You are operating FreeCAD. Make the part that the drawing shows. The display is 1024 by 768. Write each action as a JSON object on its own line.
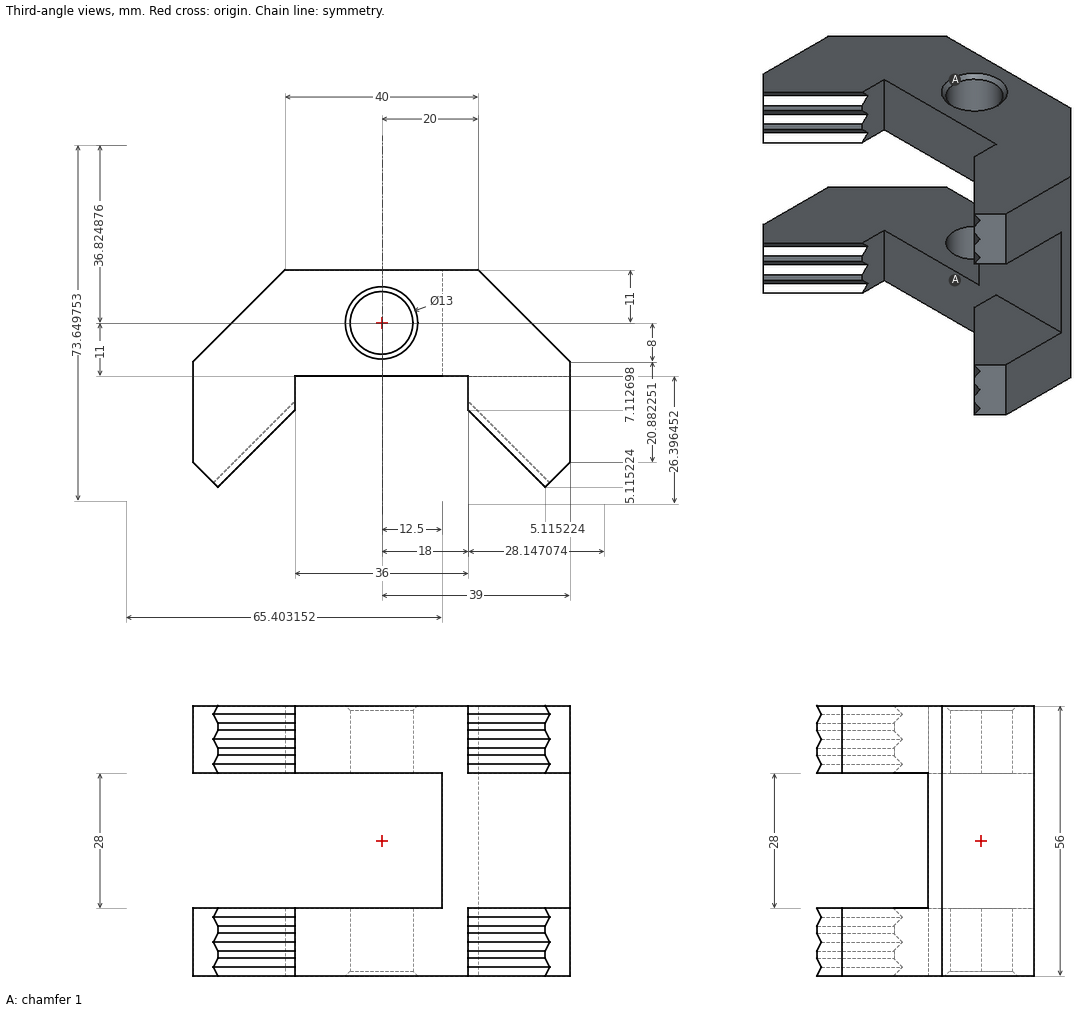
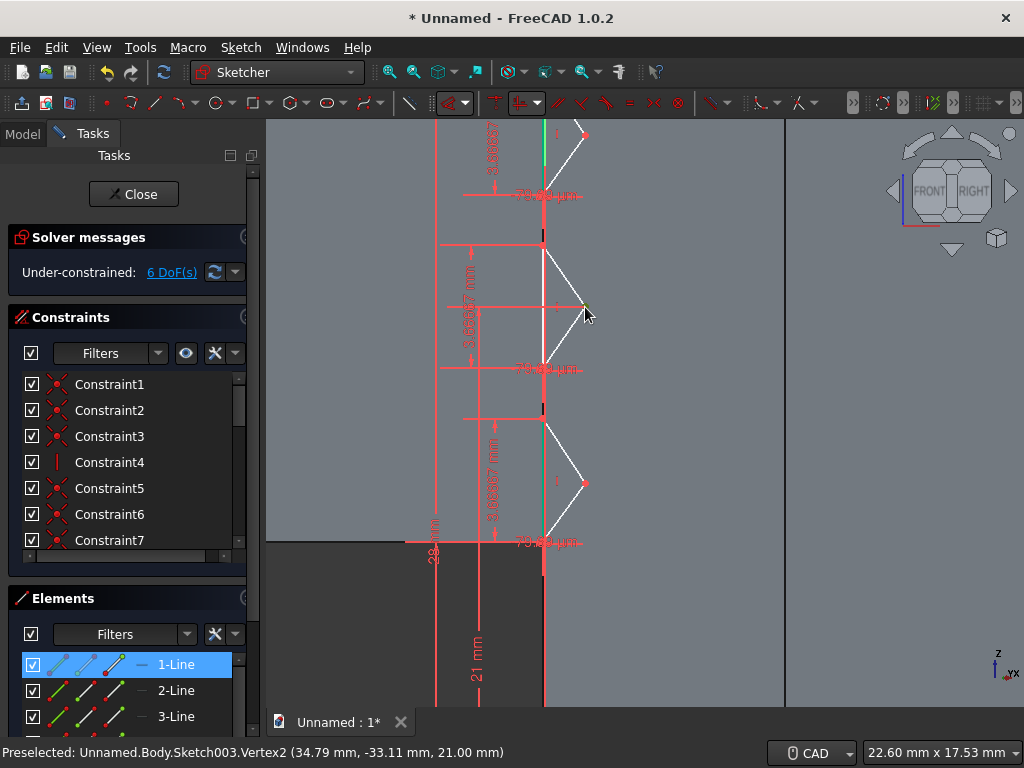
{"action": "key", "text": "l"}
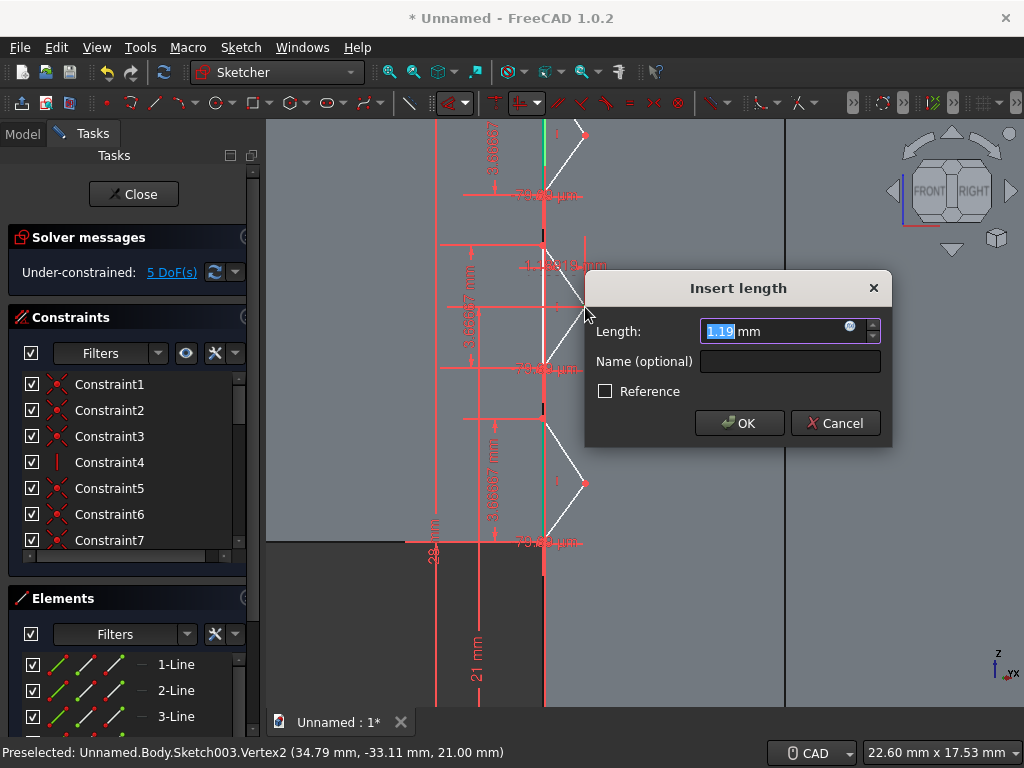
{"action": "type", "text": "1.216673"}
{"action": "key", "text": "Return"}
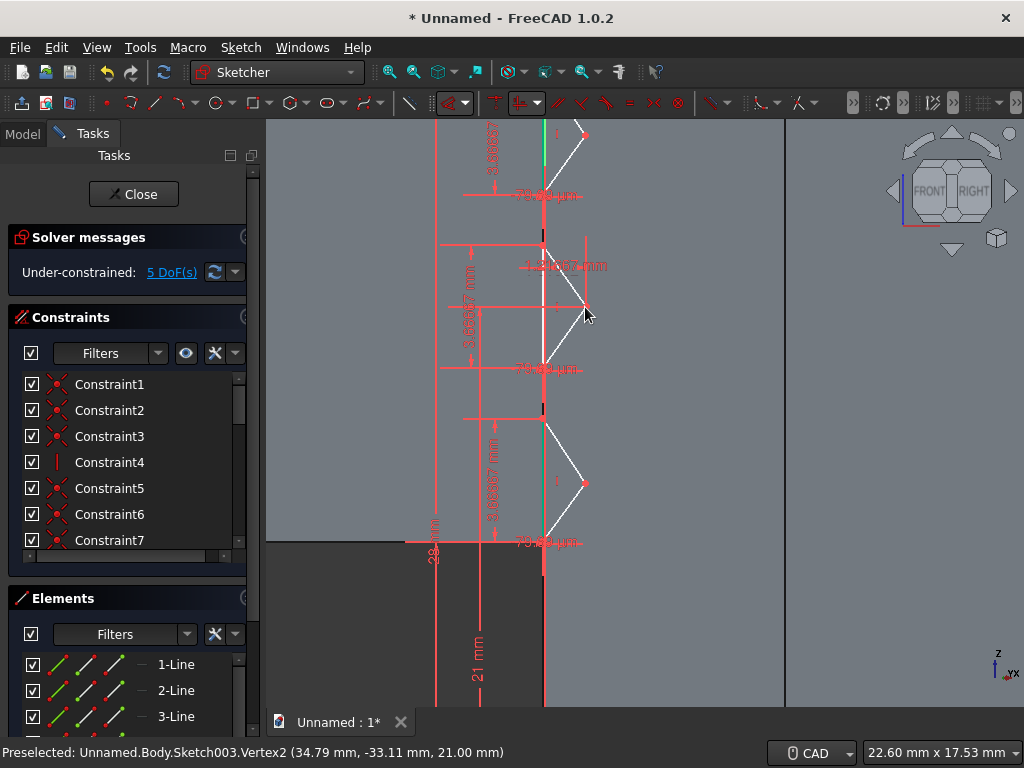
{"action": "left_click", "coordinate": [585, 483]}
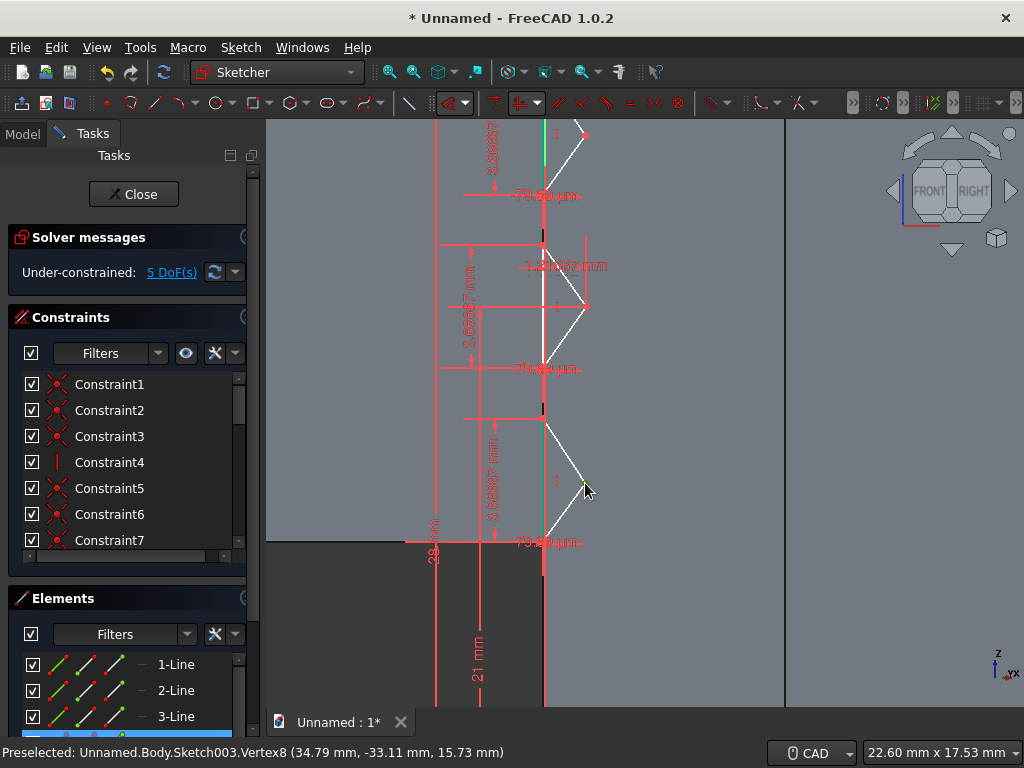
{"action": "left_click", "coordinate": [468, 104]}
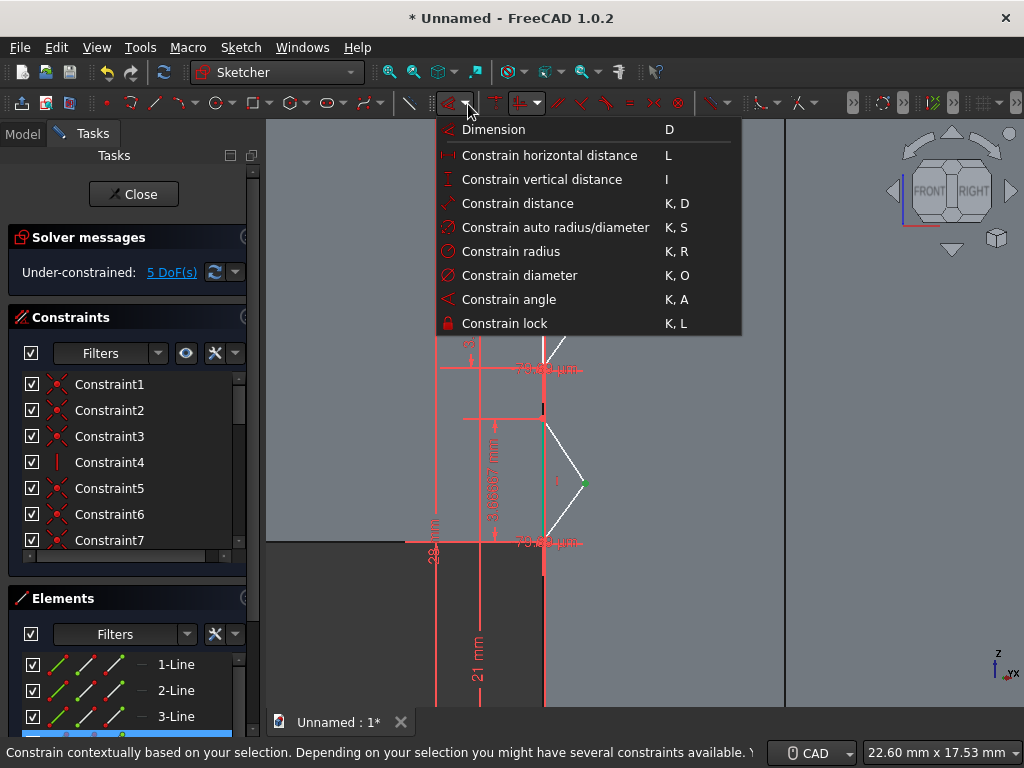
{"action": "left_click", "coordinate": [589, 155]}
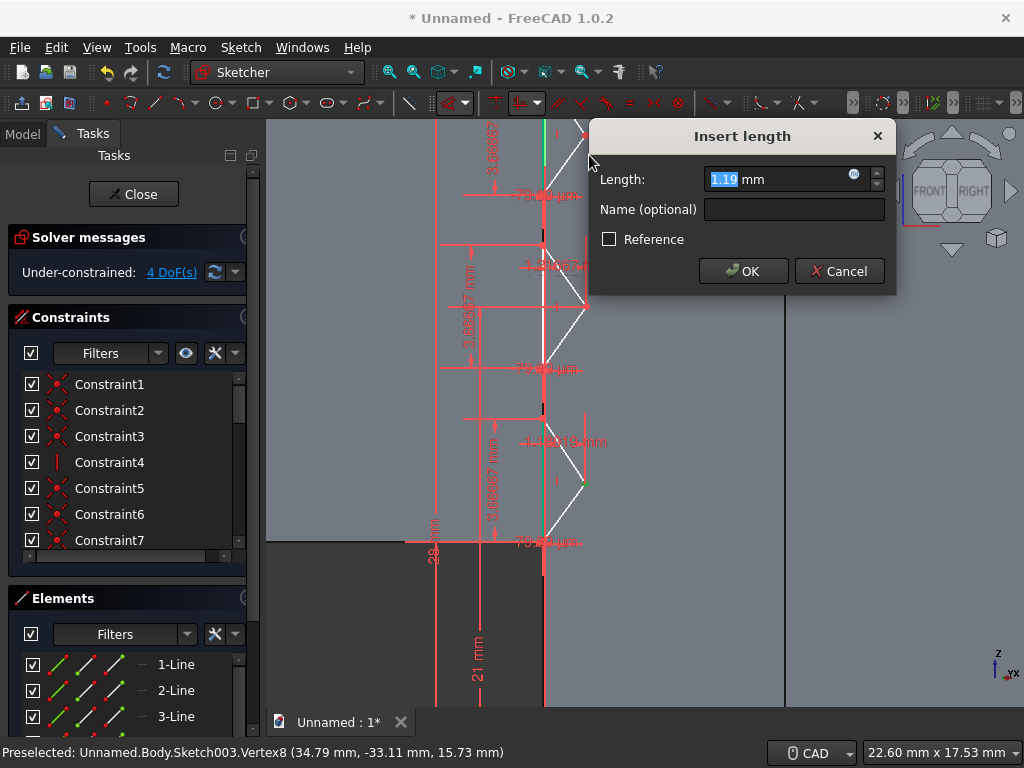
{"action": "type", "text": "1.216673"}
{"action": "key", "text": "Return"}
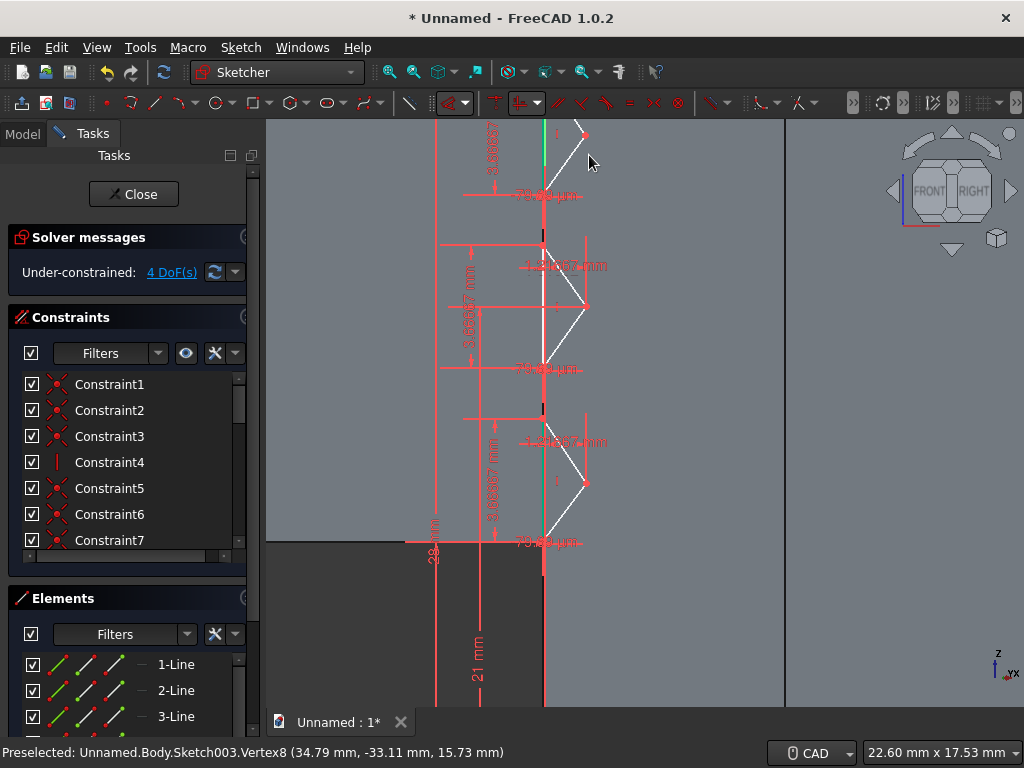
{"action": "scroll", "coordinate": [583, 338], "scroll_direction": "down", "scroll_amount": 5}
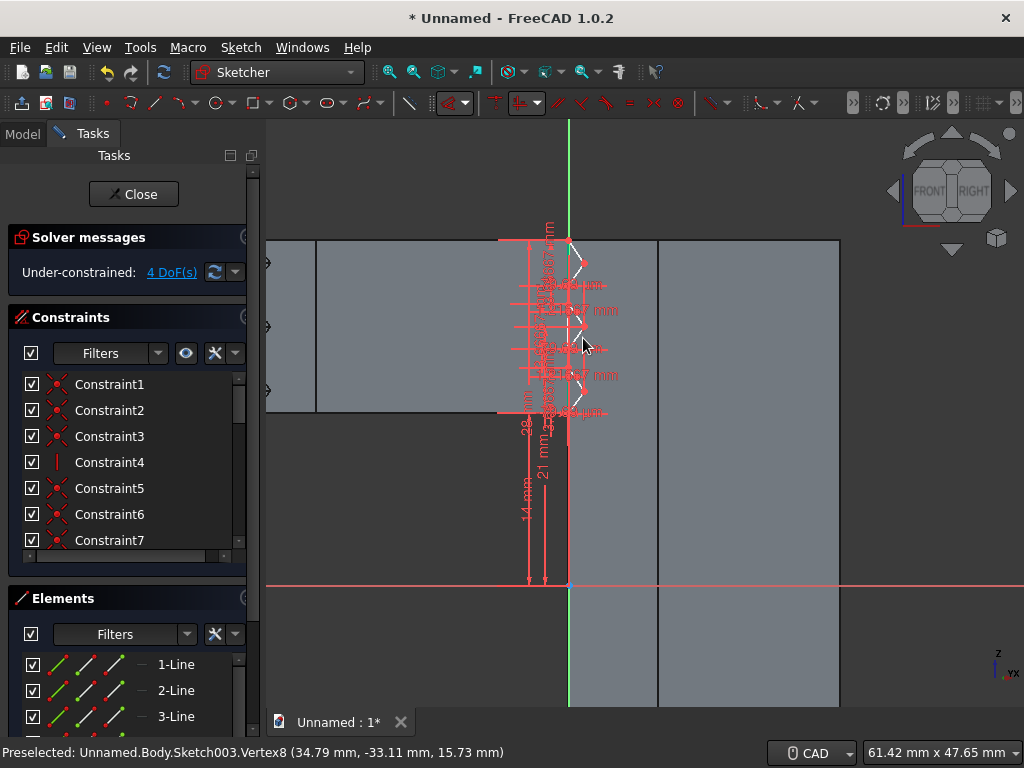
{"action": "scroll", "coordinate": [584, 264], "scroll_direction": "up", "scroll_amount": 5}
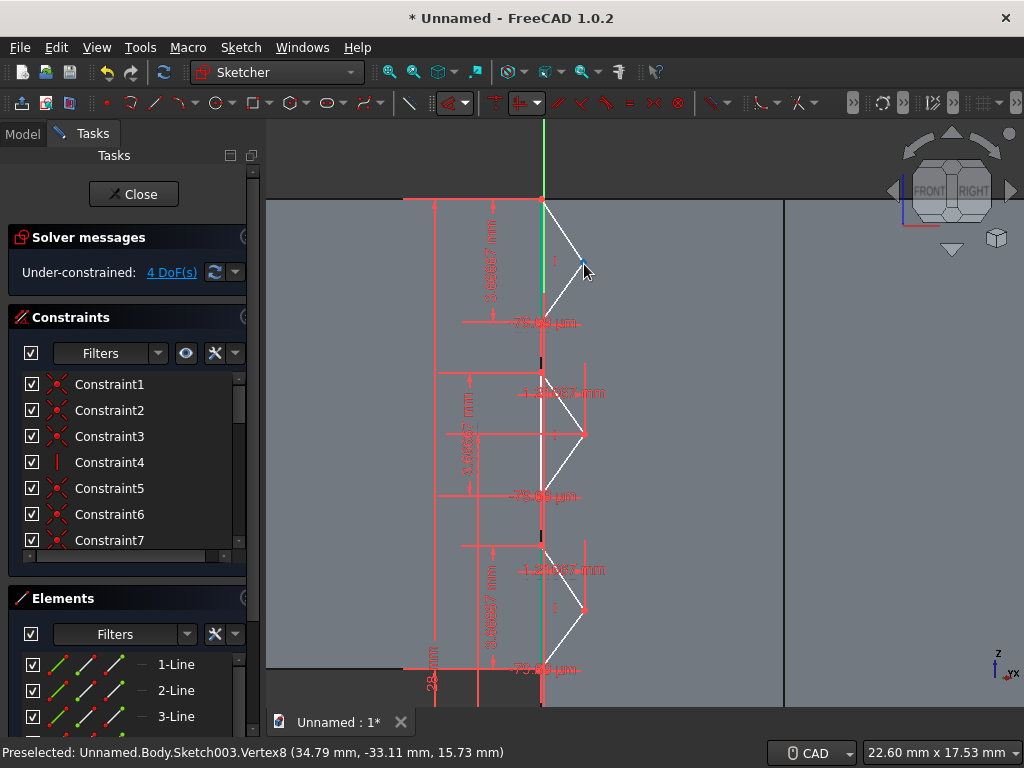
{"action": "left_click", "coordinate": [584, 263]}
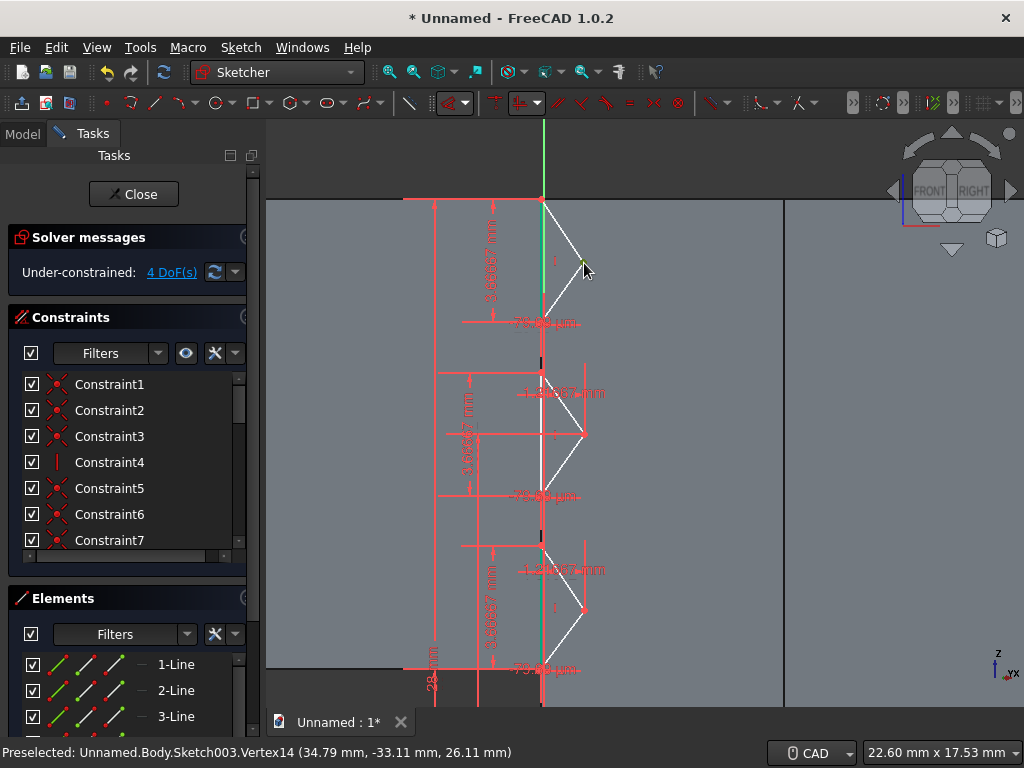
{"action": "key", "text": "l"}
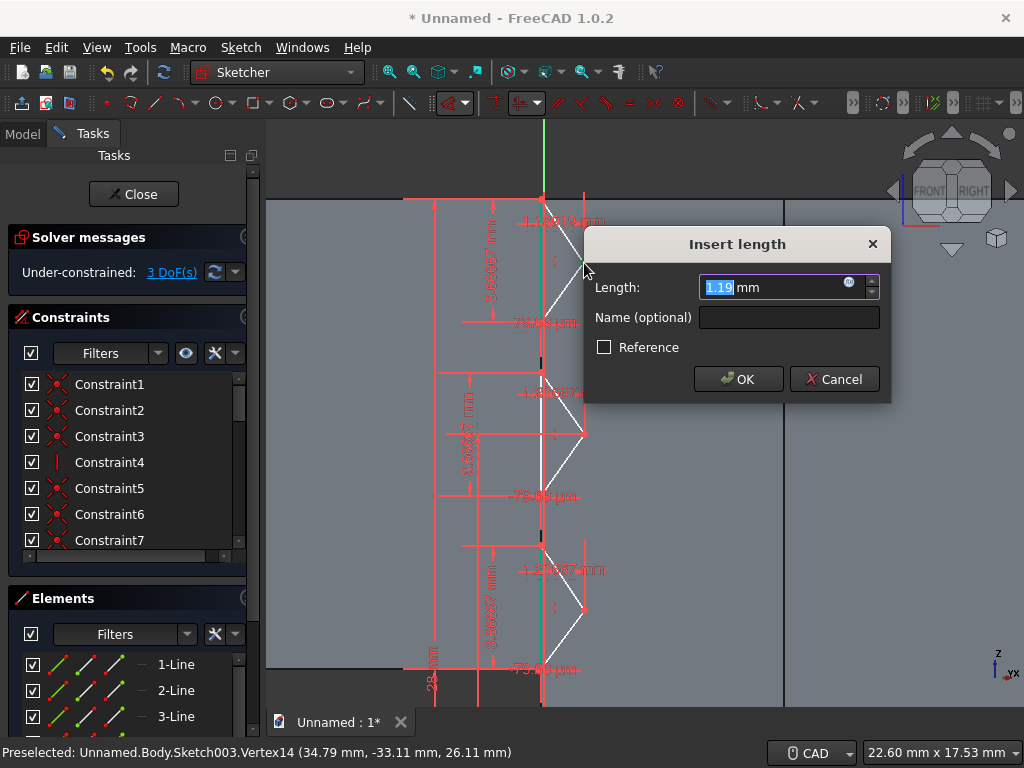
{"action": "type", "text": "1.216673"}
{"action": "key", "text": "Return"}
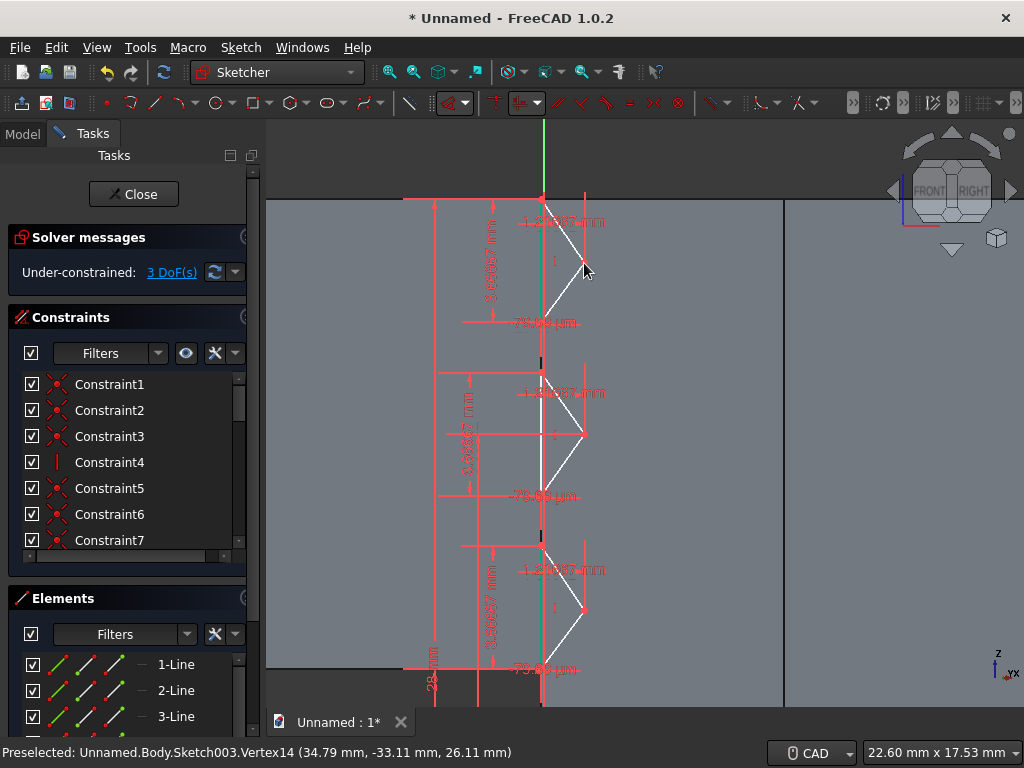
{"action": "scroll", "coordinate": [554, 477], "scroll_direction": "up", "scroll_amount": 2}